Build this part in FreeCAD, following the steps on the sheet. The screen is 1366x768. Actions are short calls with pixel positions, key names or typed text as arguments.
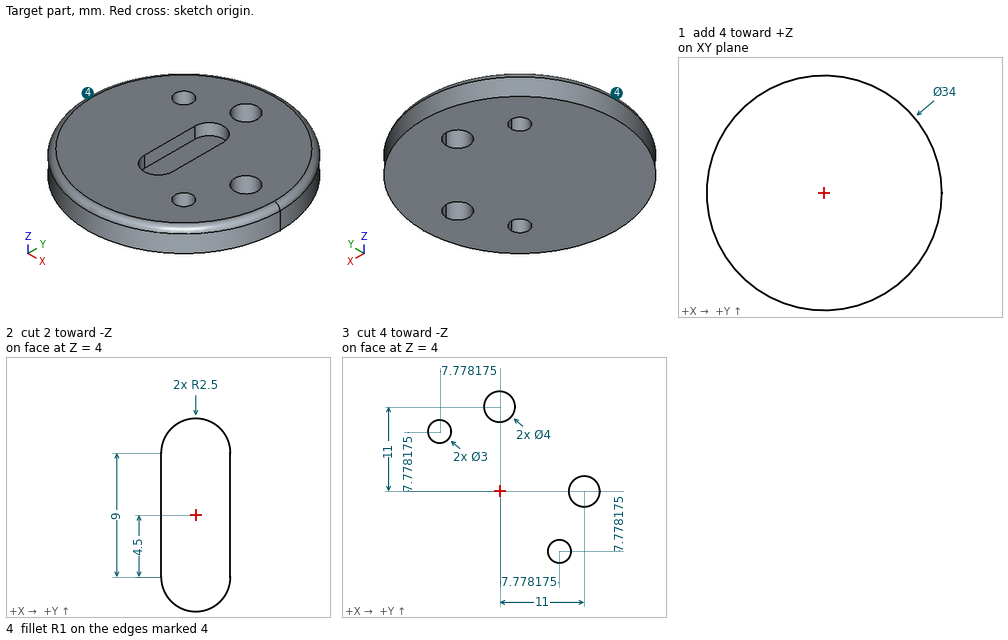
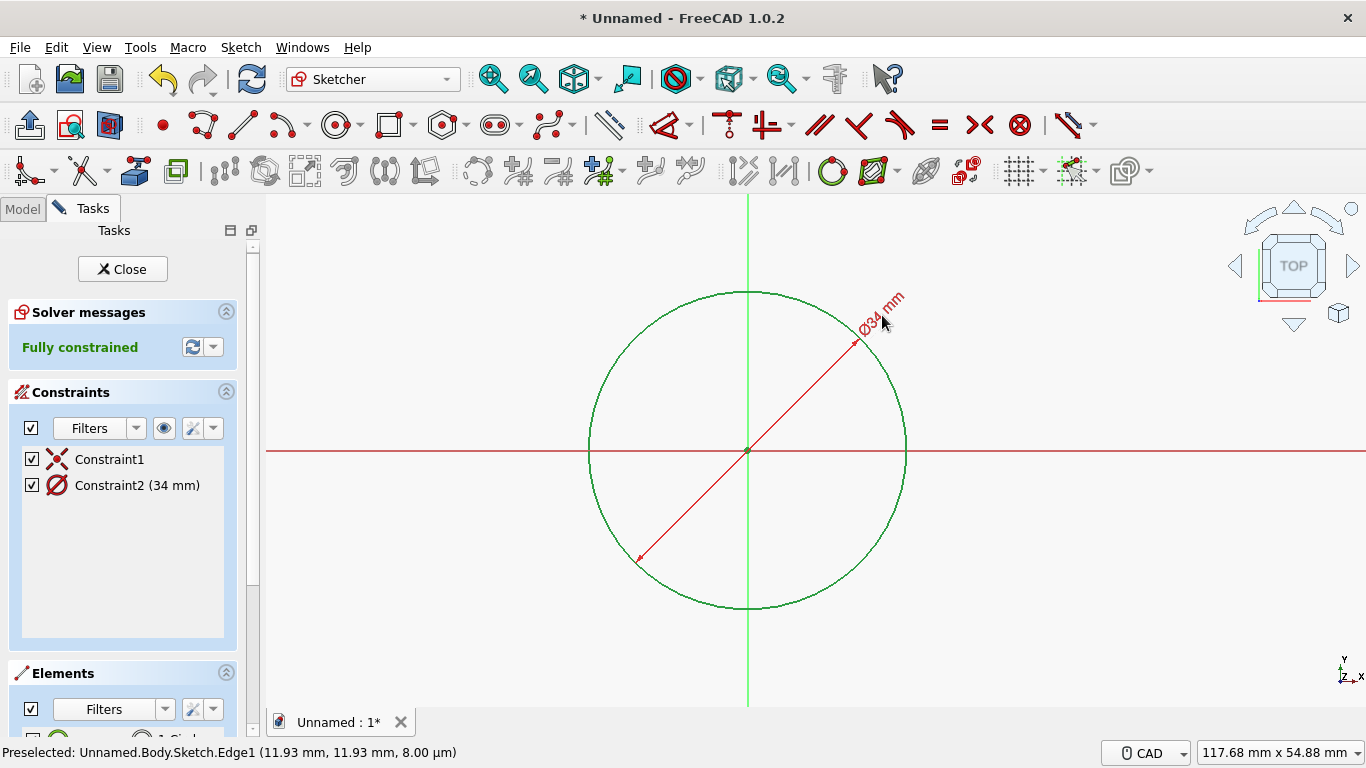
click(123, 269)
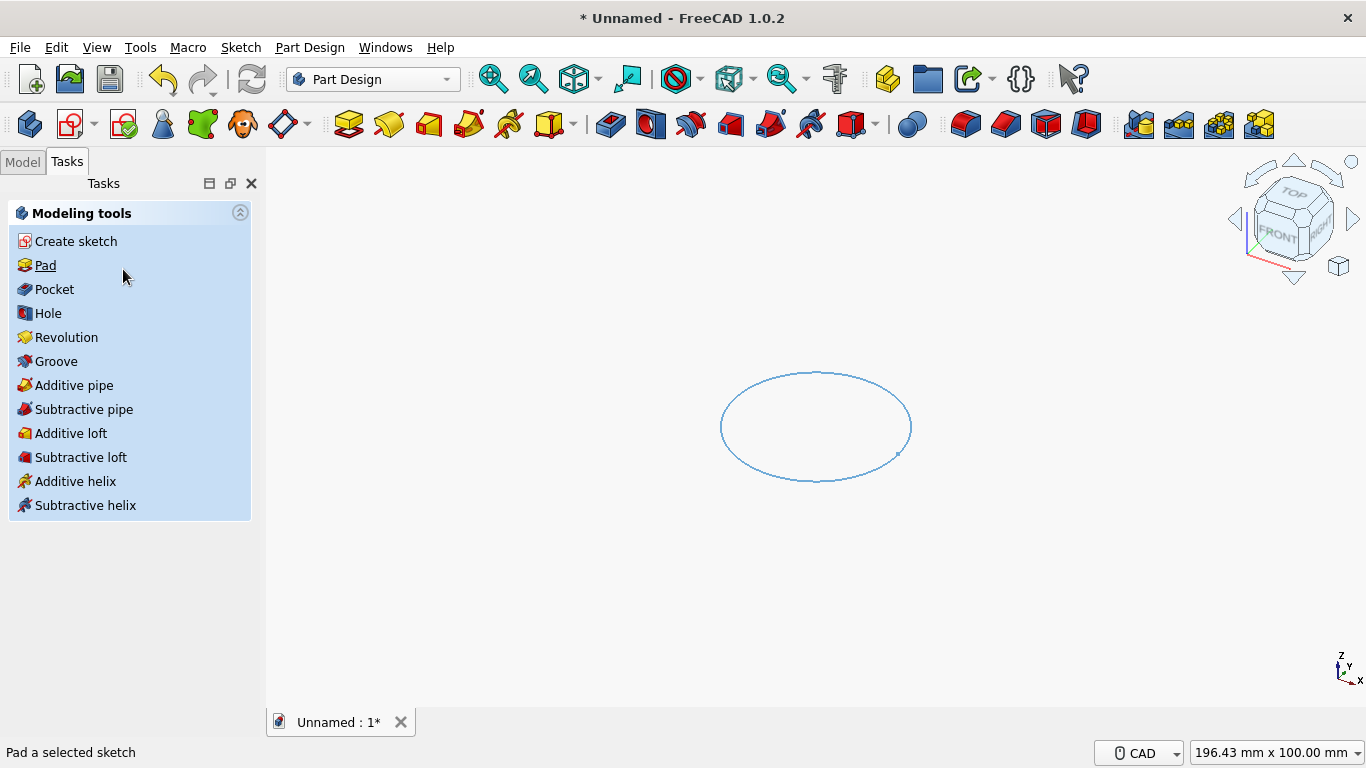
click(350, 124)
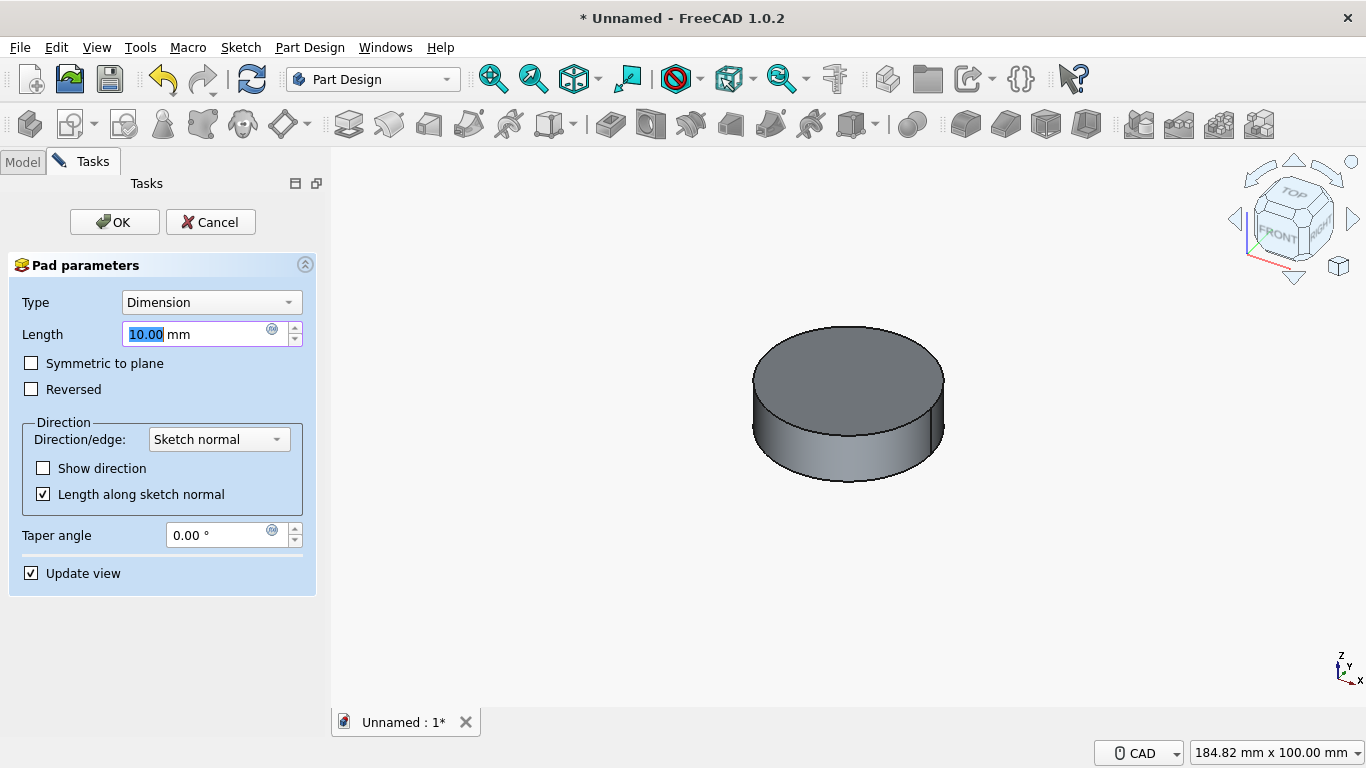
text(4)
key(Tab)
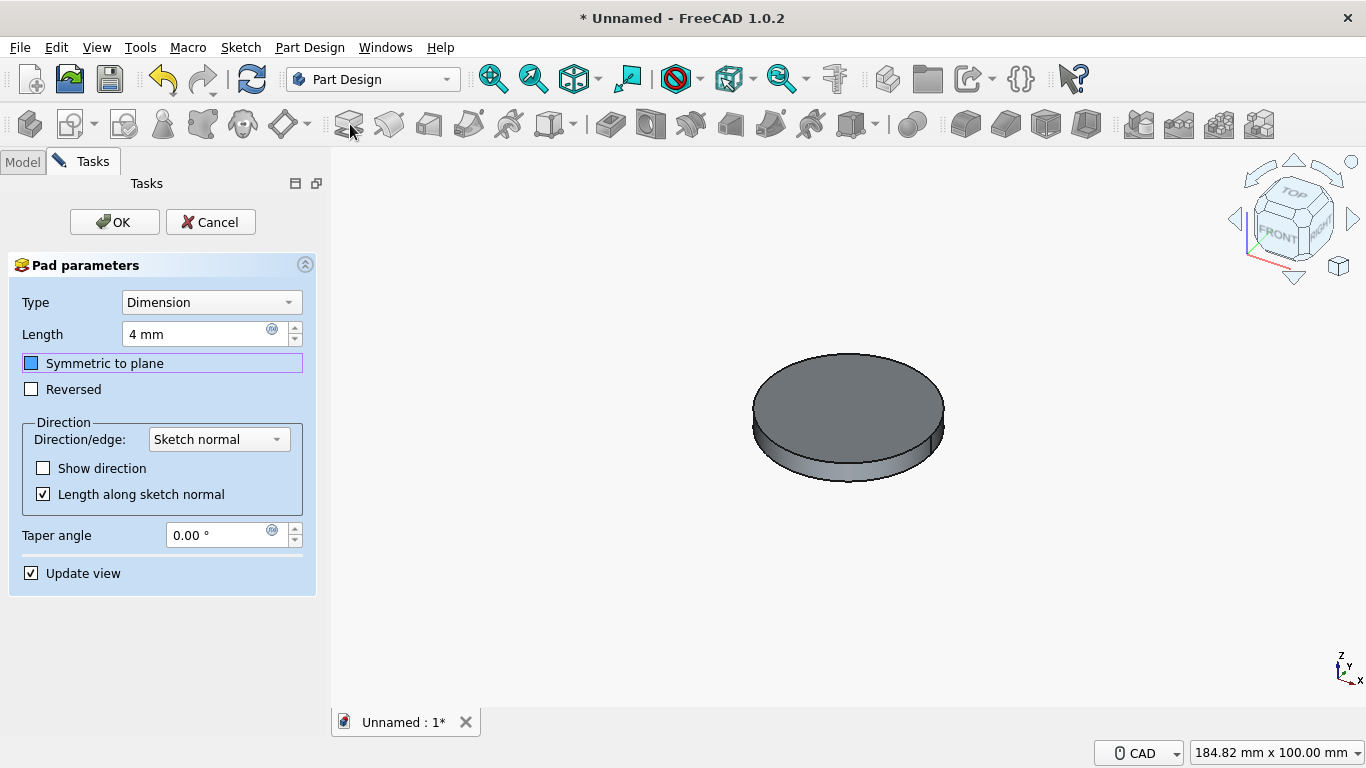
click(115, 222)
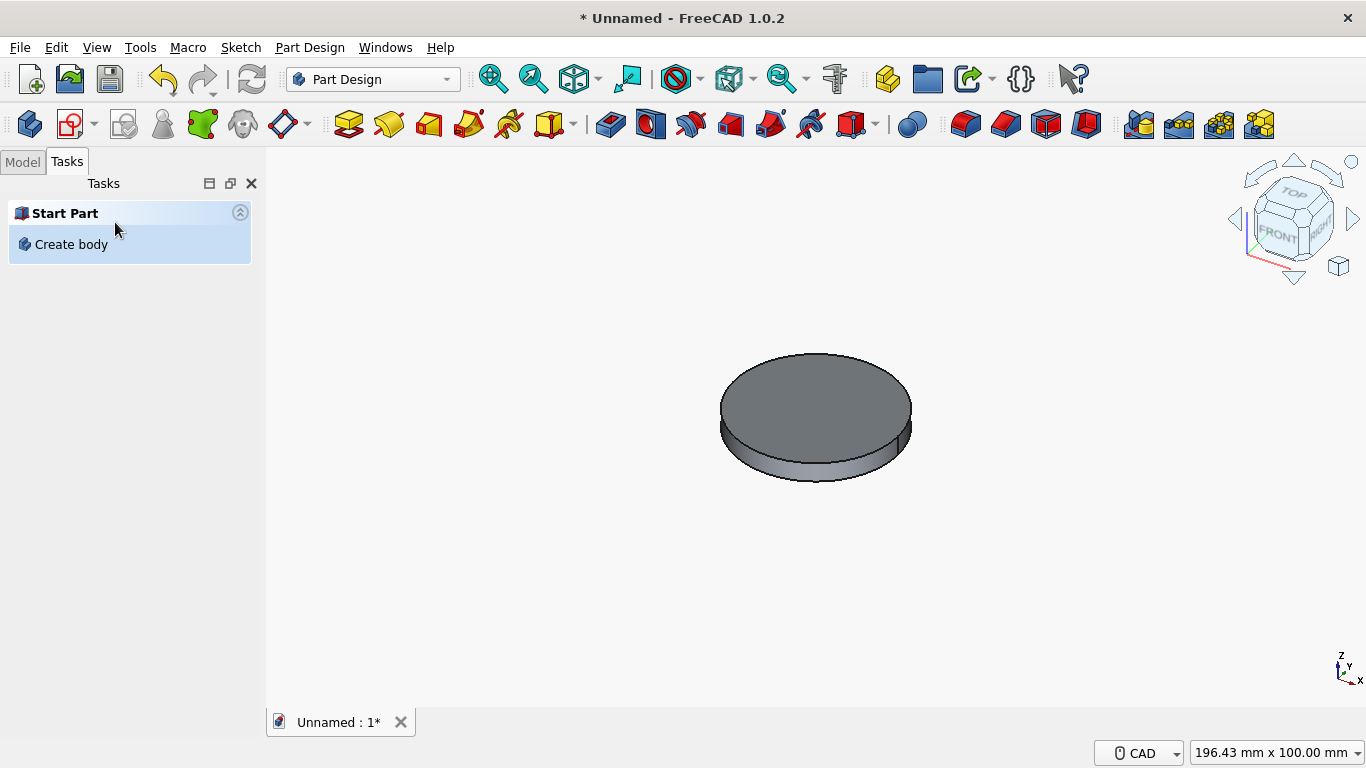
key(v)
key(f)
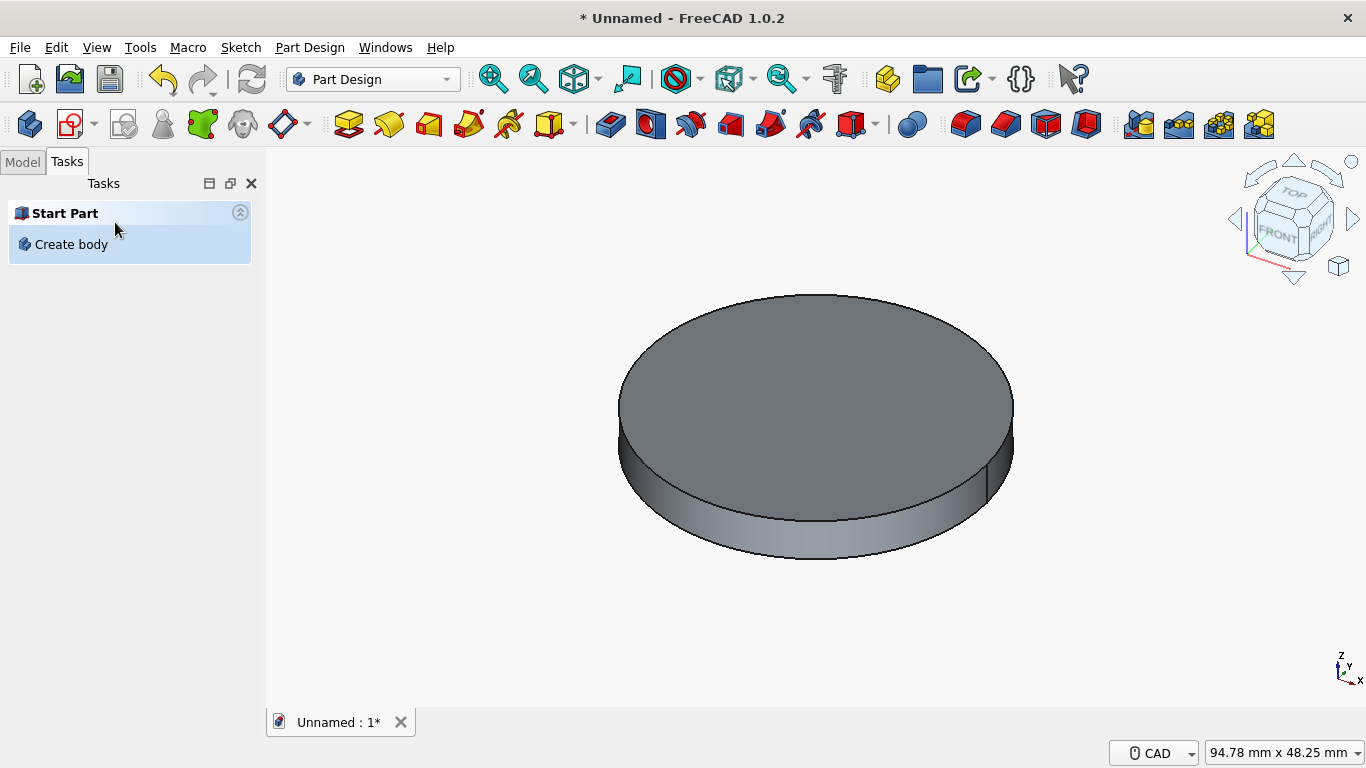
click(816, 407)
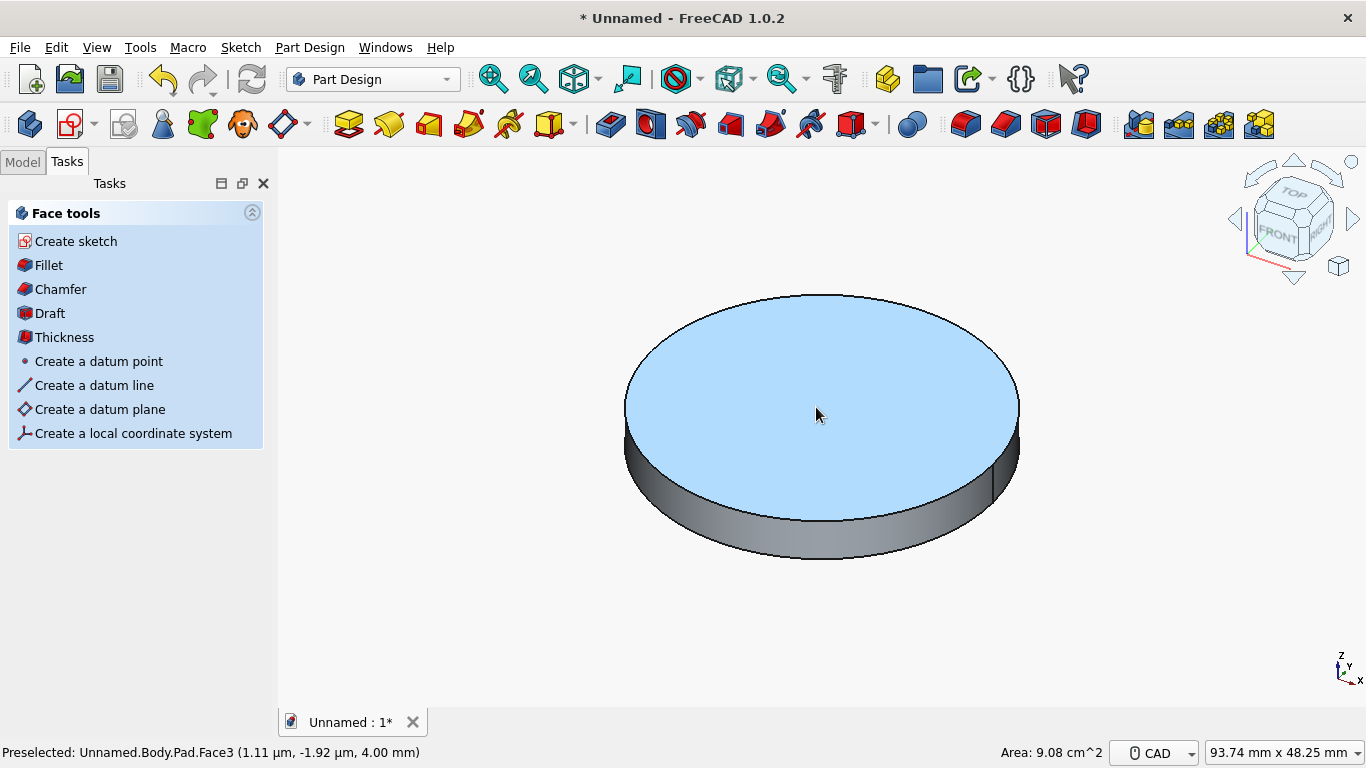
click(70, 124)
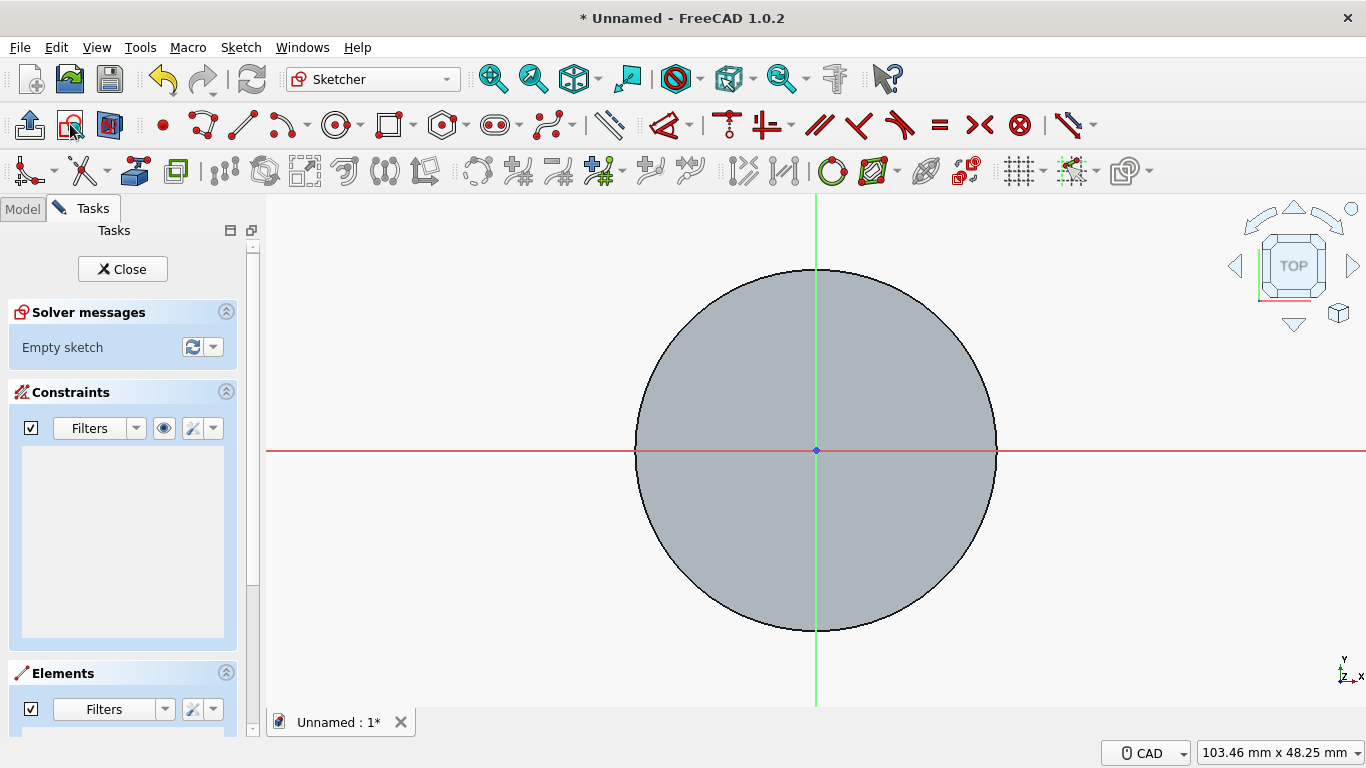
scroll(872, 450, up, 4)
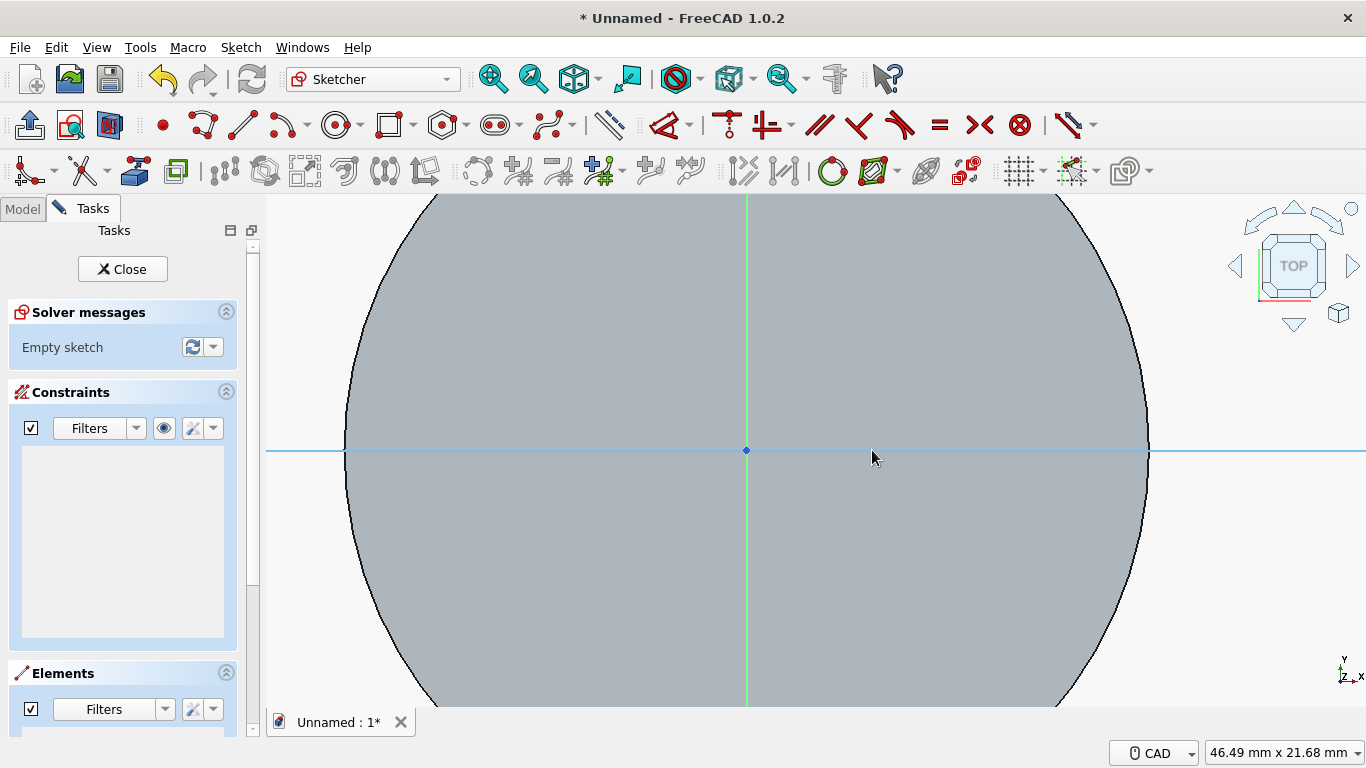
click(496, 126)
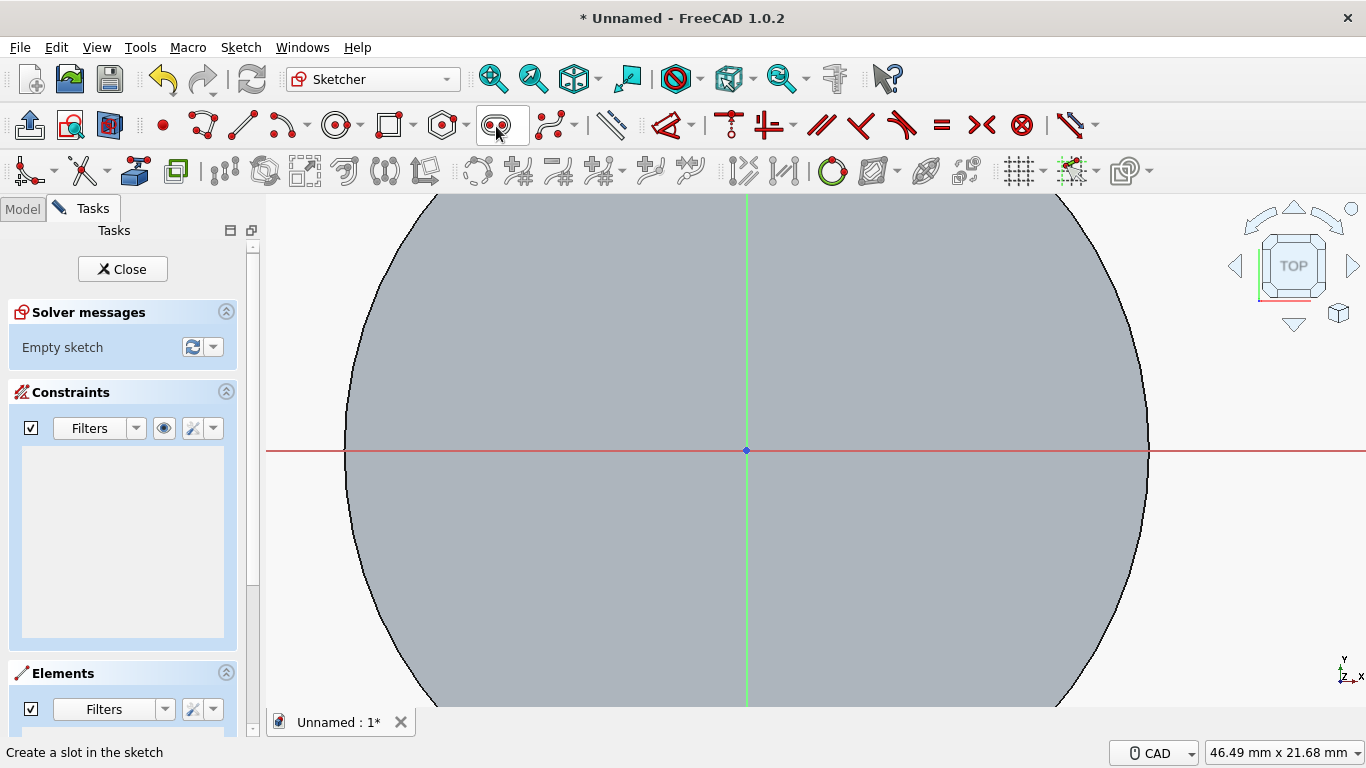
click(747, 557)